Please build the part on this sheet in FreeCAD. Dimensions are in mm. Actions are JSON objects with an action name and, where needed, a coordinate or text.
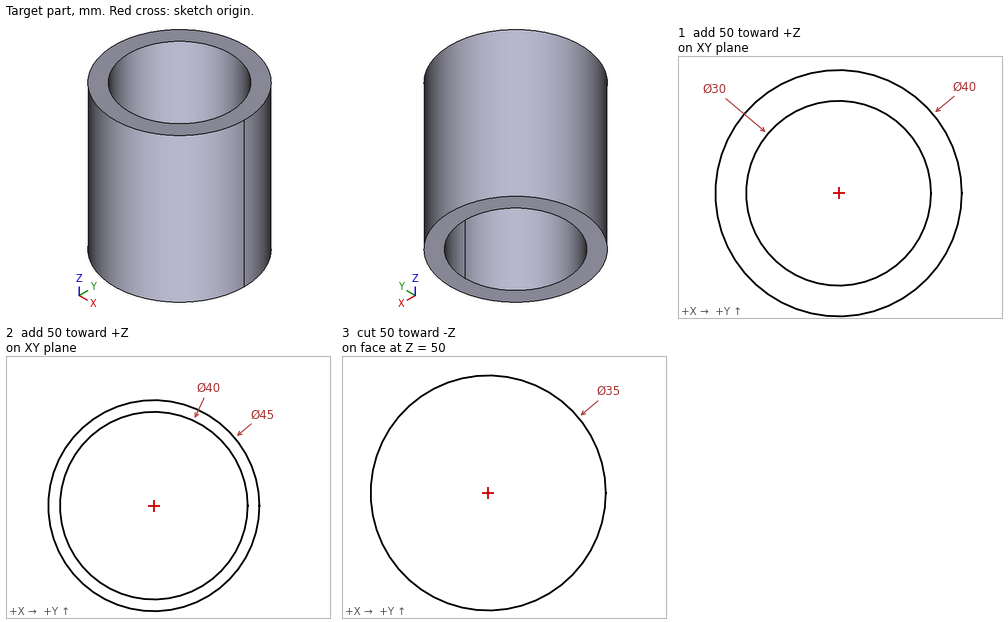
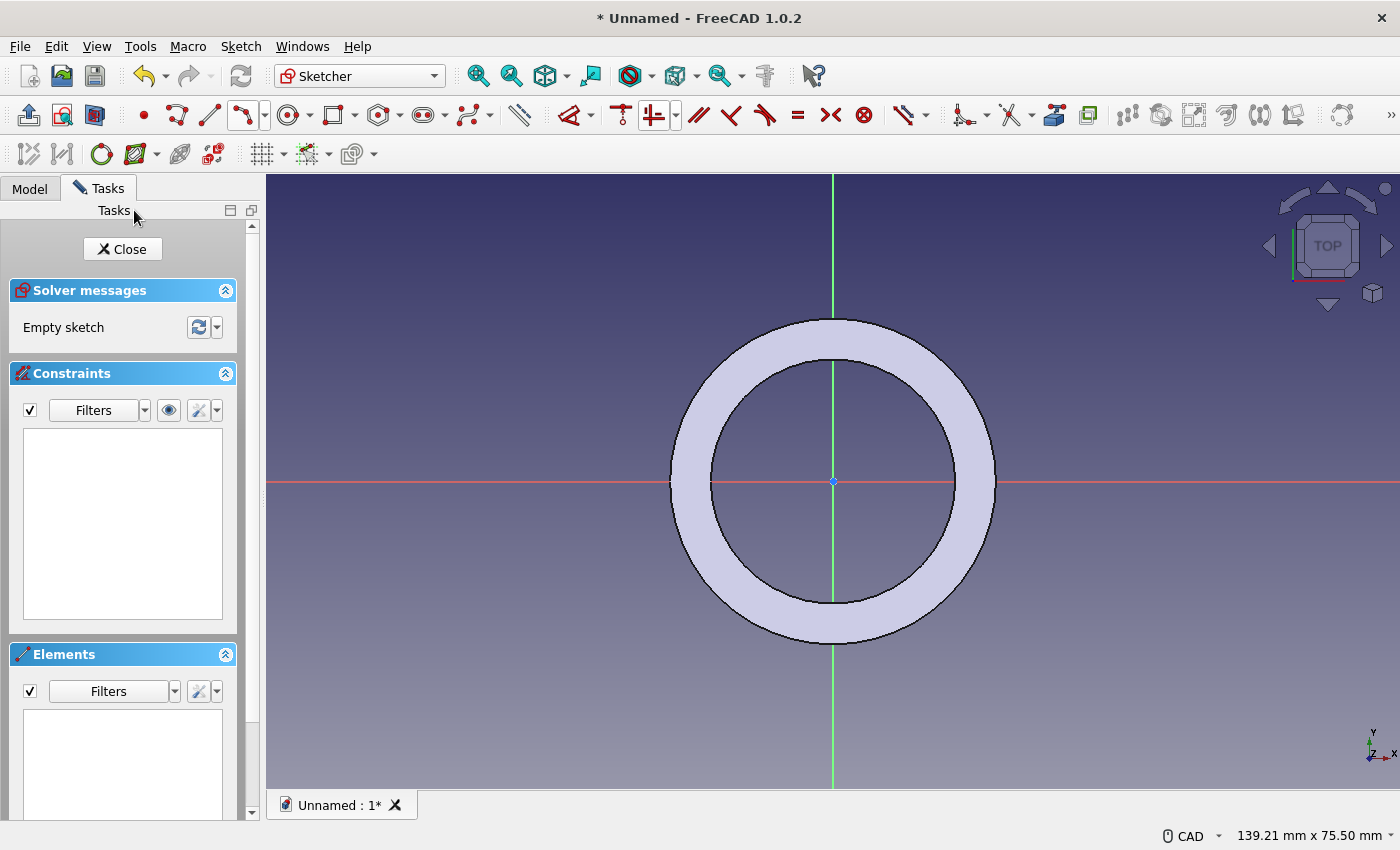
{"action": "left_click", "coordinate": [95, 116]}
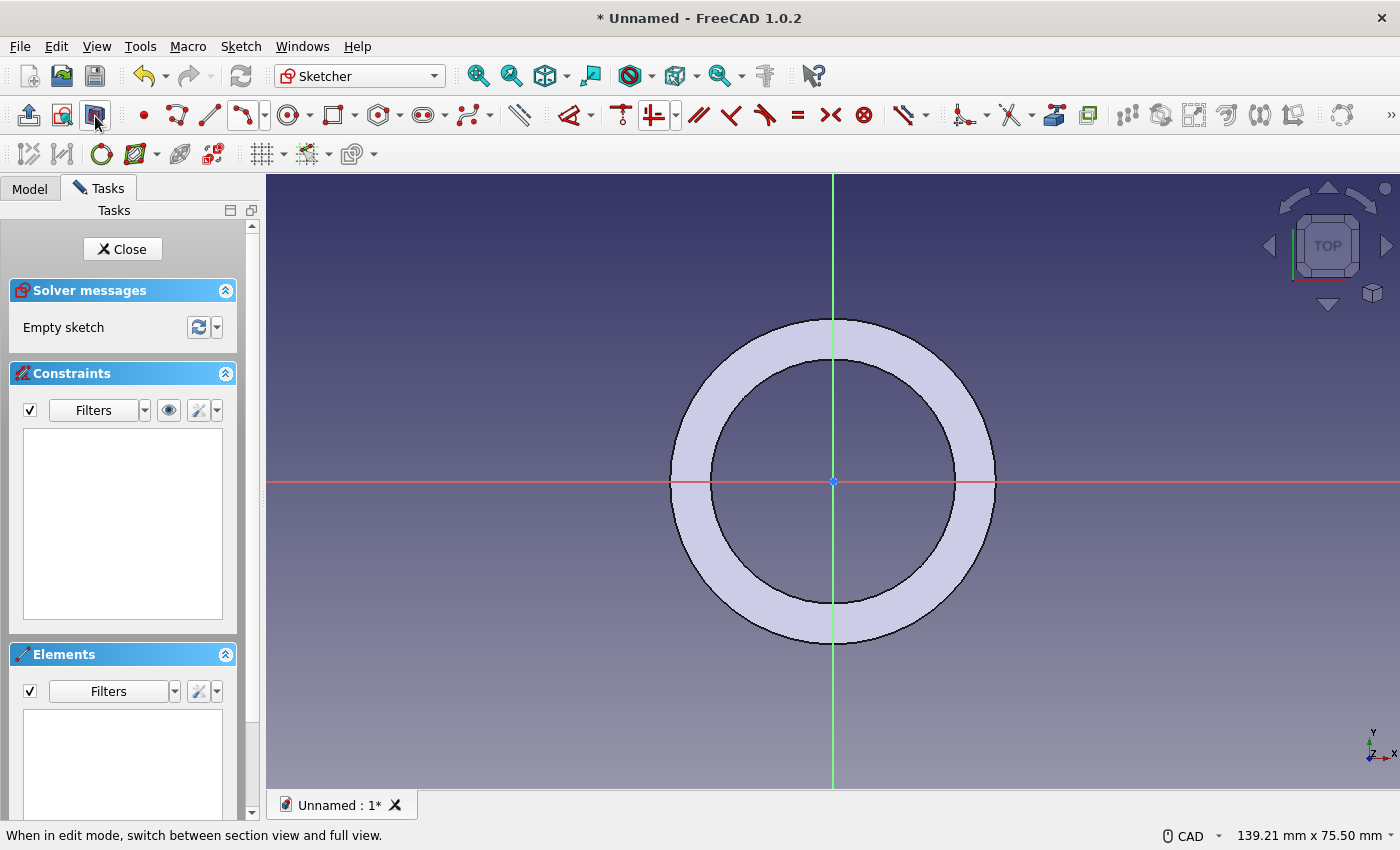
{"action": "key", "text": "g c"}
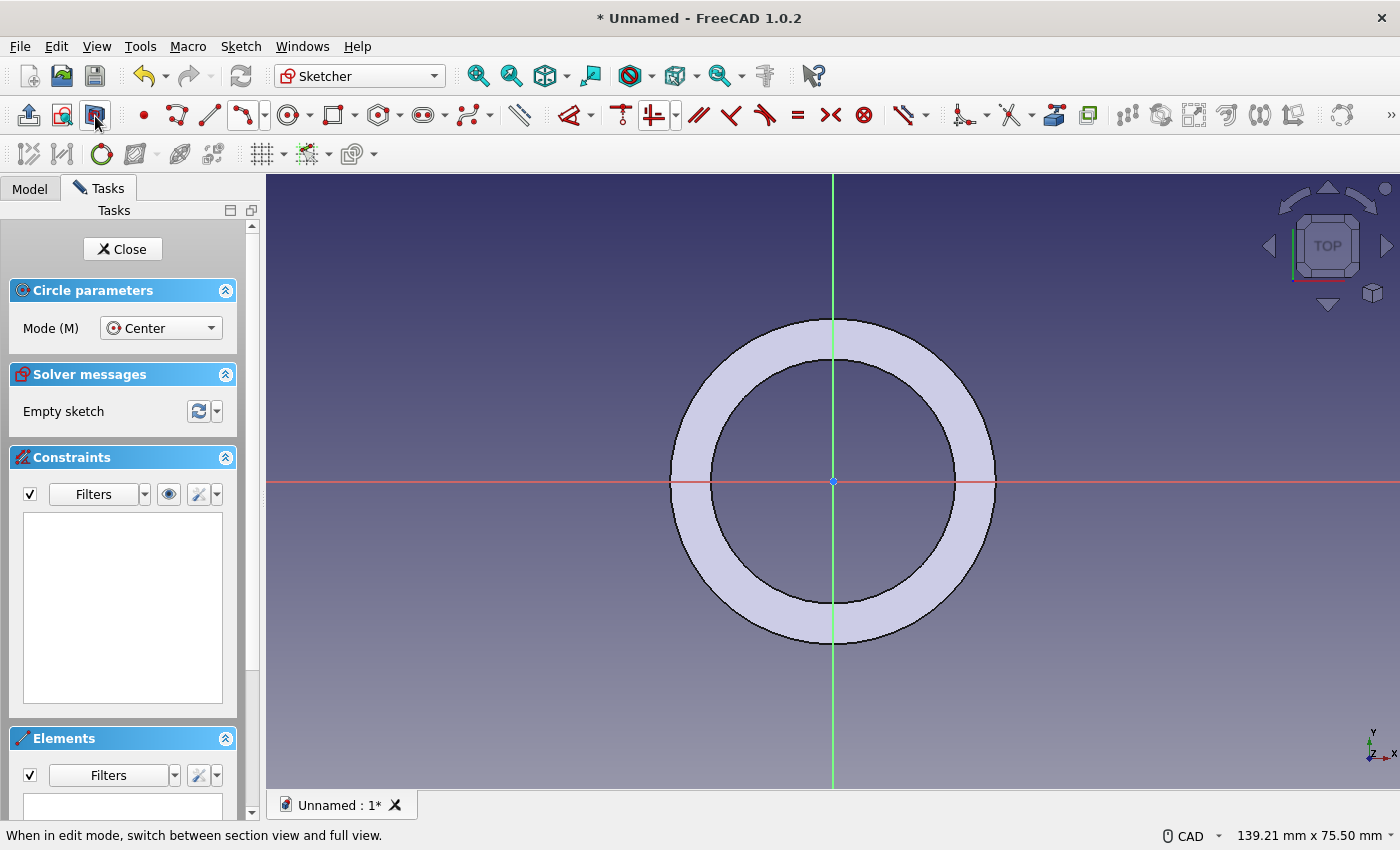
{"action": "left_click", "coordinate": [833, 482]}
{"action": "mouse_move", "coordinate": [963, 352]}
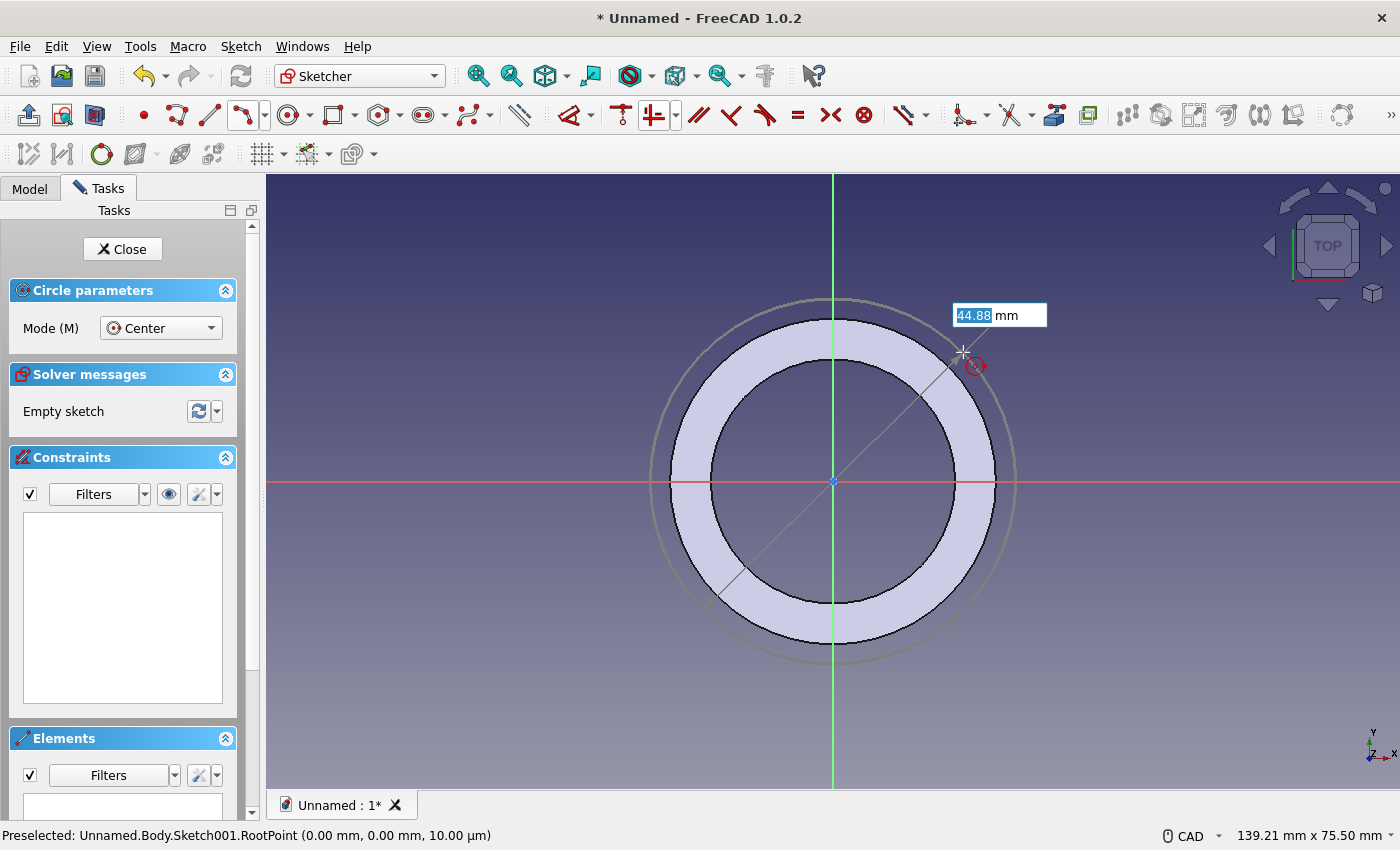
{"action": "type", "text": "45"}
{"action": "key", "text": "Return"}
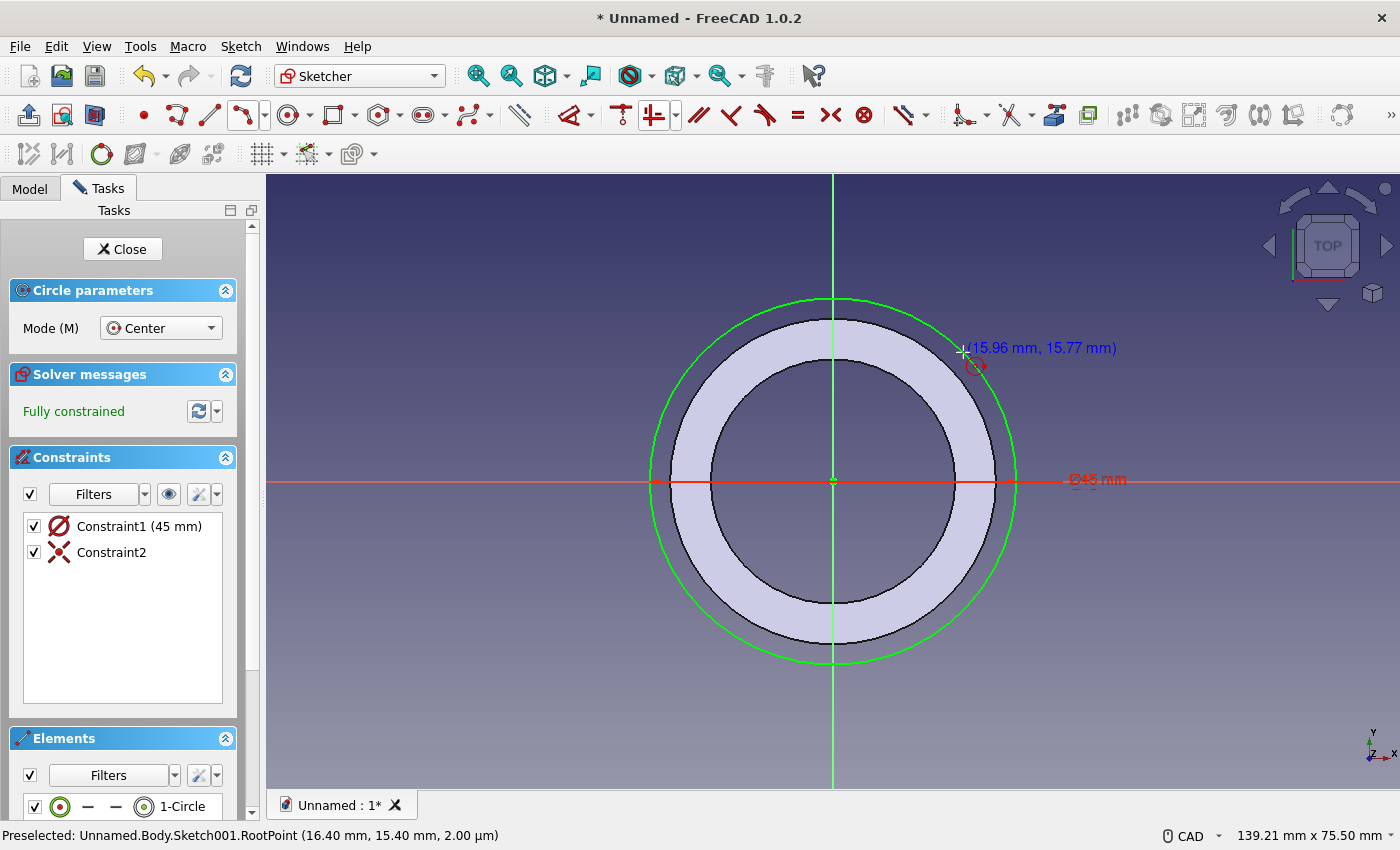
{"action": "left_click", "coordinate": [833, 482]}
{"action": "mouse_move", "coordinate": [948, 366]}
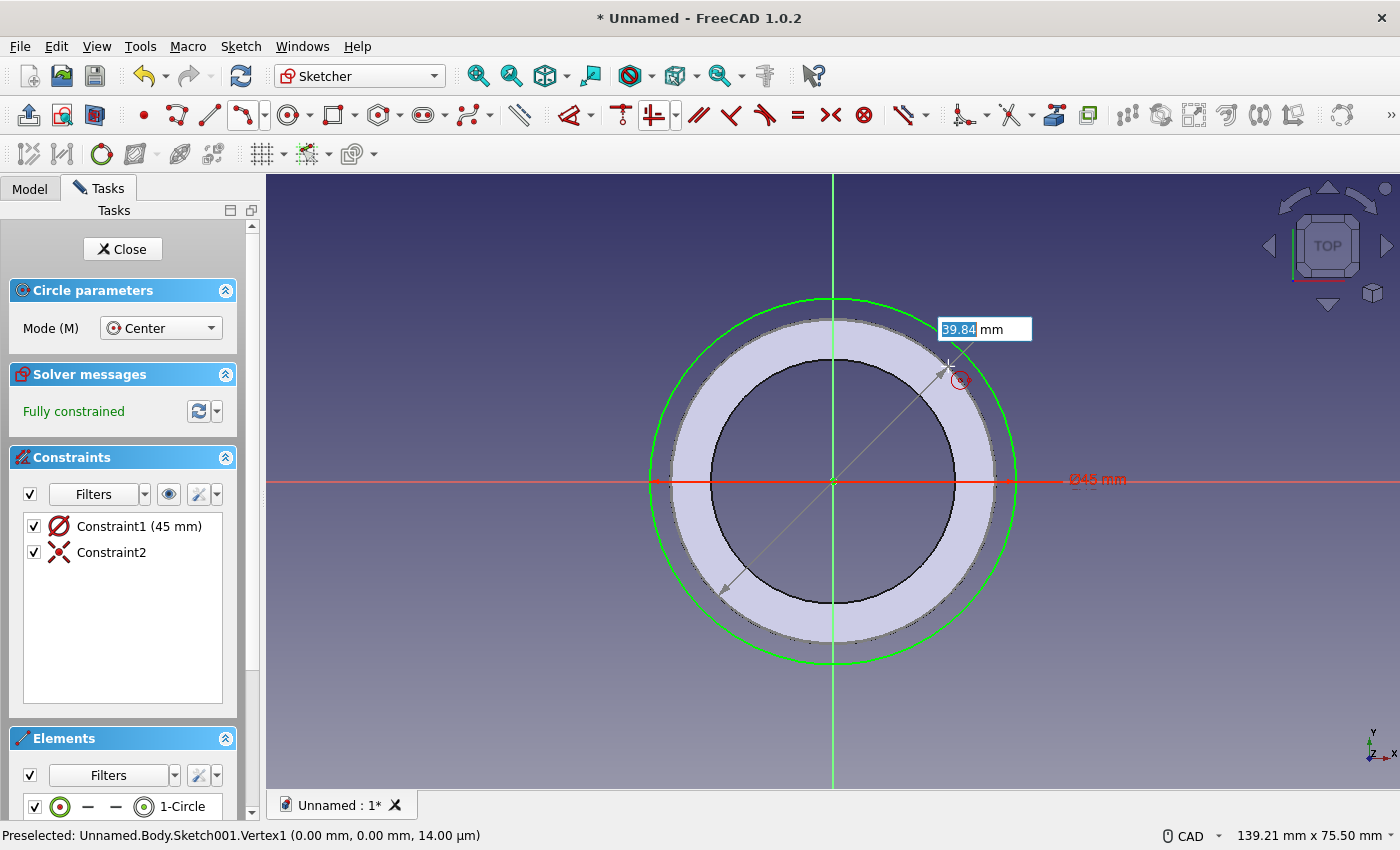
{"action": "type", "text": "40"}
{"action": "key", "text": "Return"}
{"action": "key", "text": "Escape"}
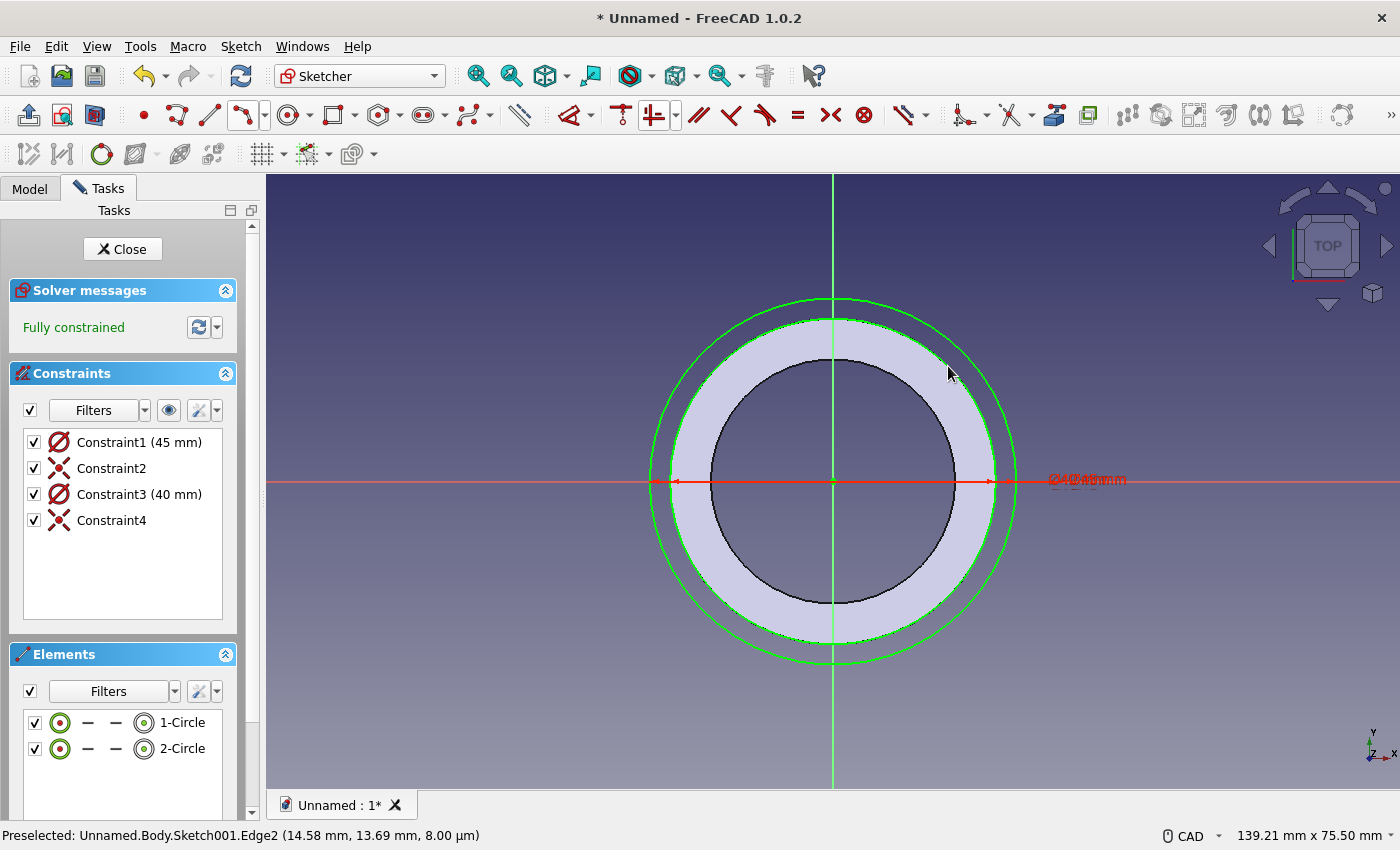
{"action": "left_click", "coordinate": [123, 249]}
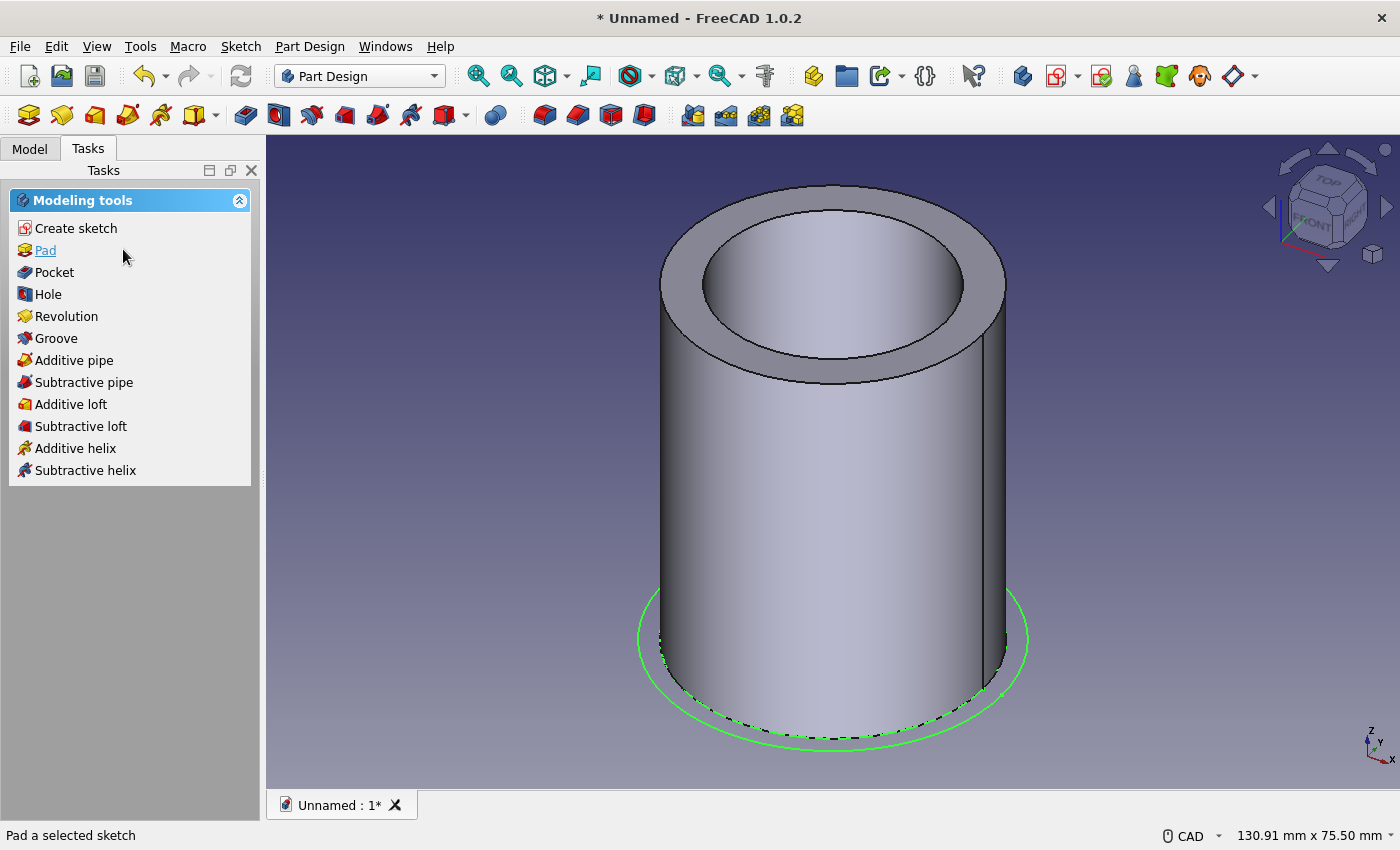
{"action": "left_click", "coordinate": [29, 116]}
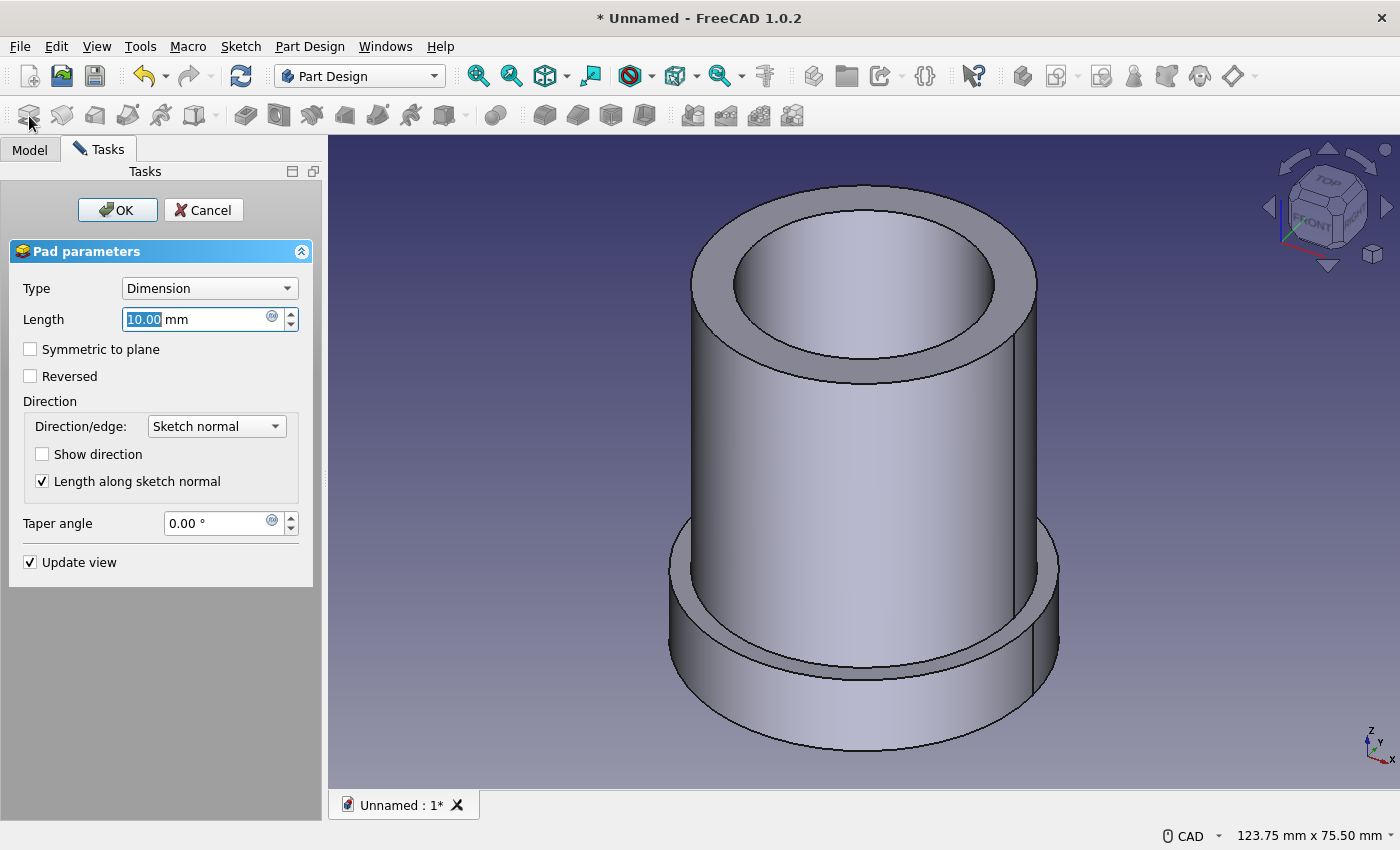
{"action": "type", "text": "50"}
{"action": "key", "text": "Tab"}